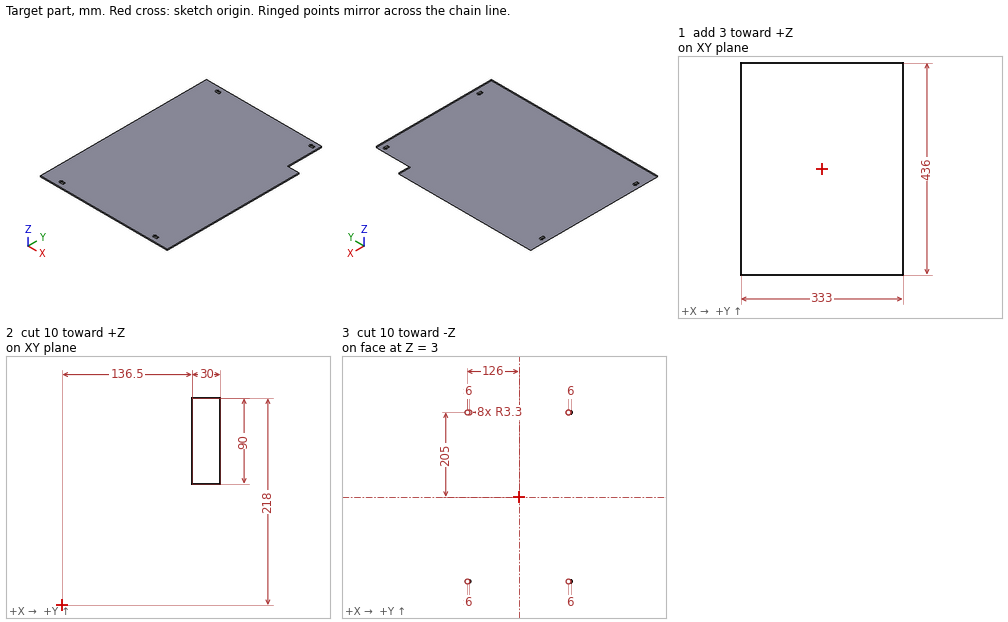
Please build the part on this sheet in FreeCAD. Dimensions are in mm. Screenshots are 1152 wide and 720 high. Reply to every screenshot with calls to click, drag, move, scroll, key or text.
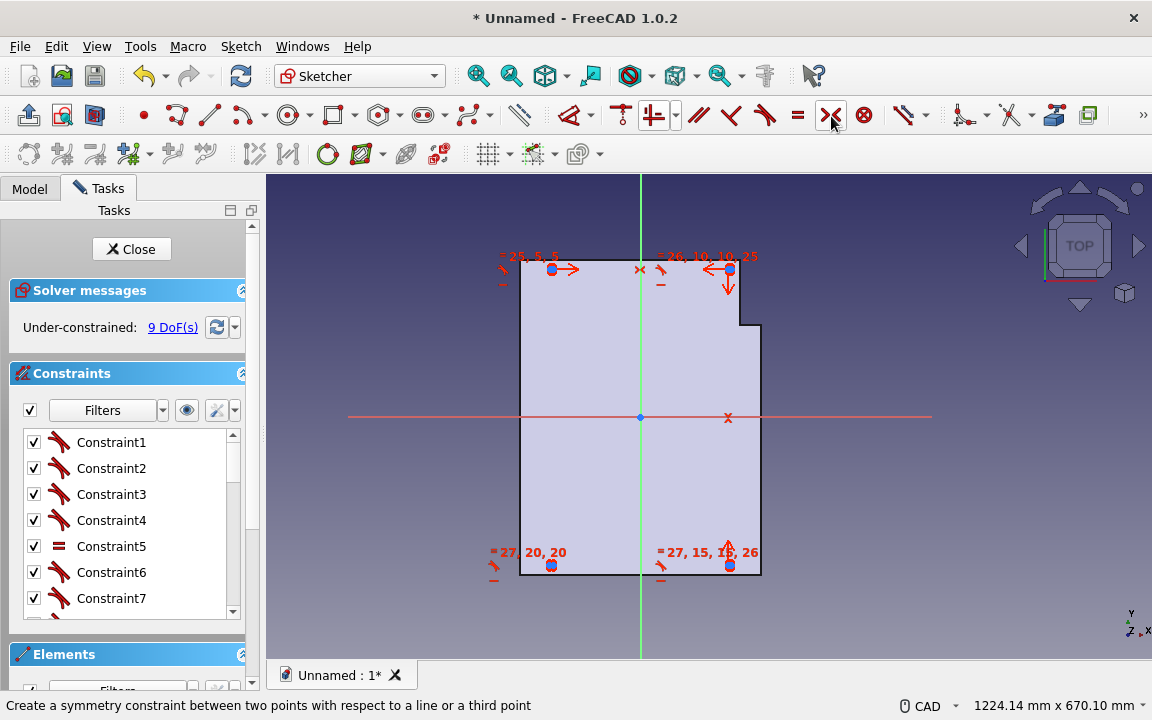
scroll(551, 269, up, 8)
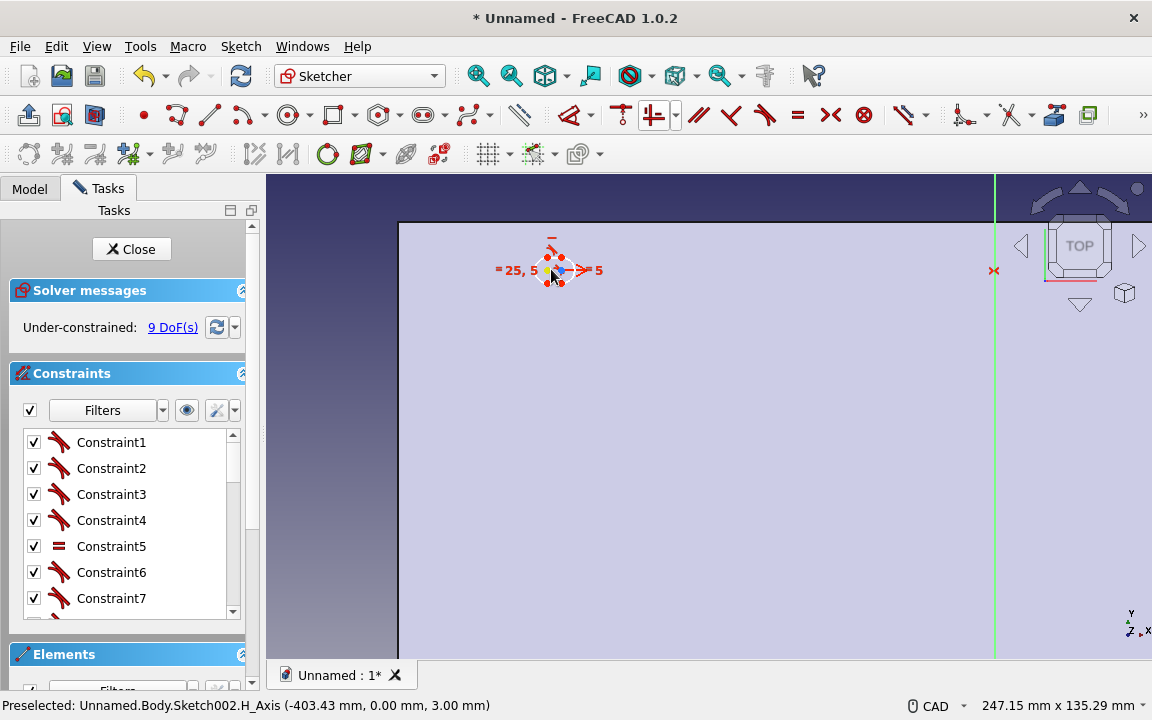
click(548, 270)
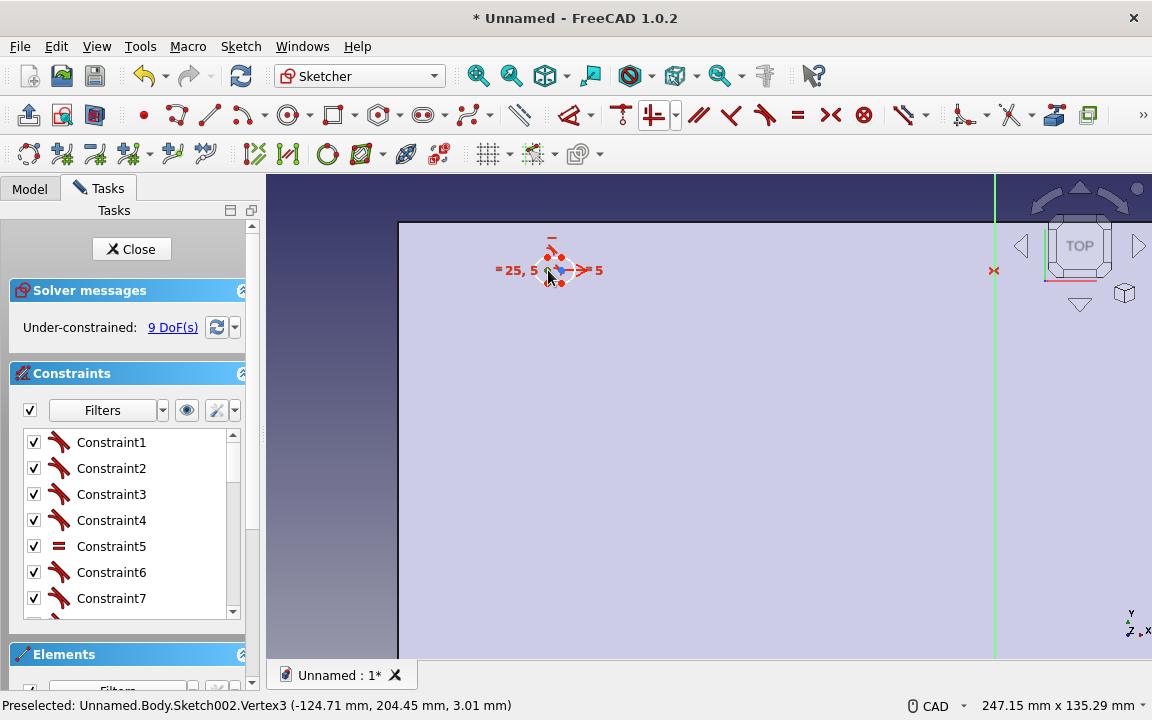
scroll(551, 268, down, 8)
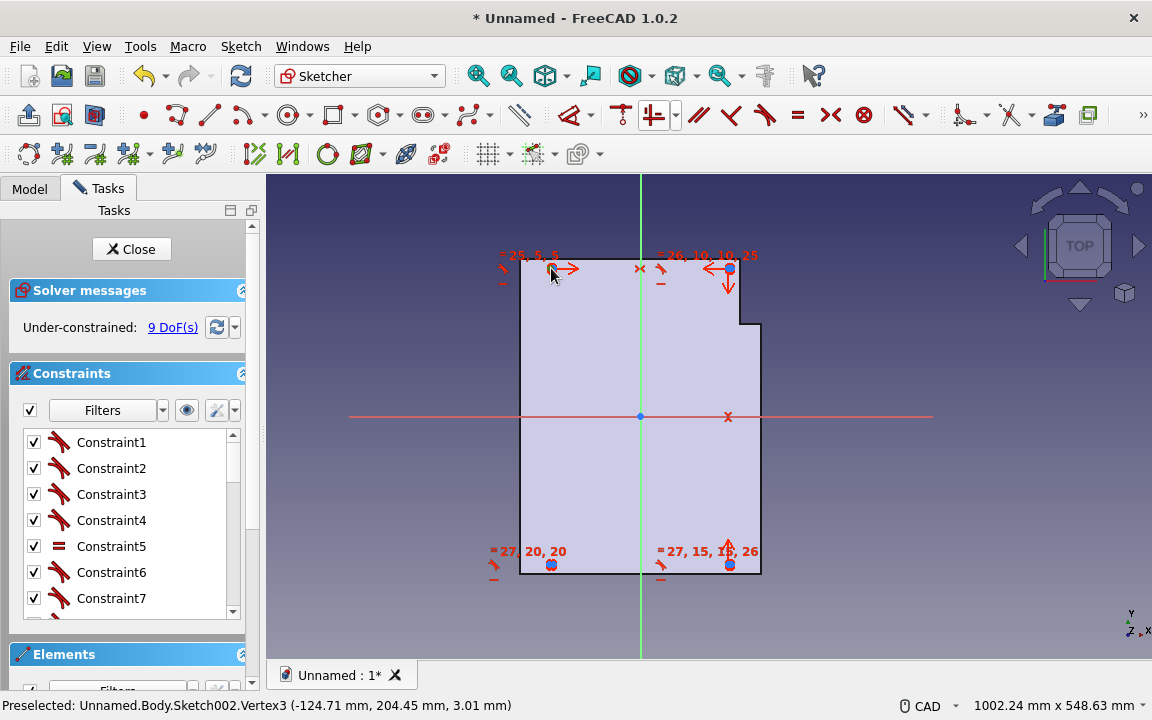
scroll(550, 565, up, 8)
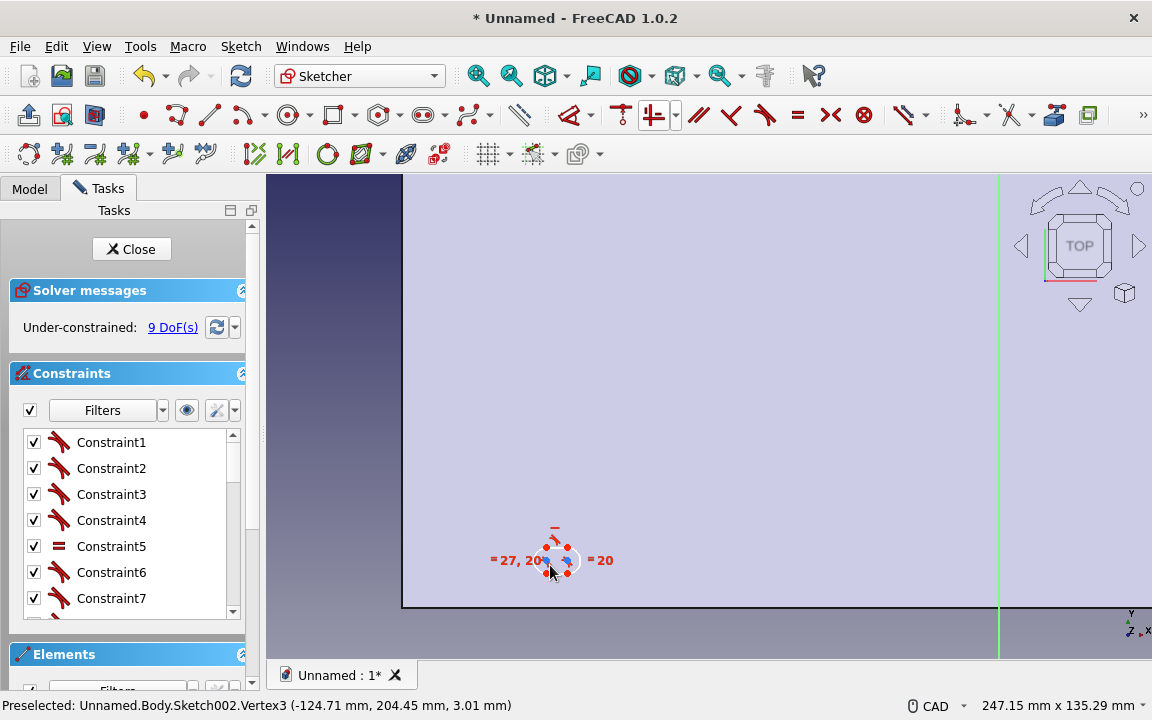
click(547, 561)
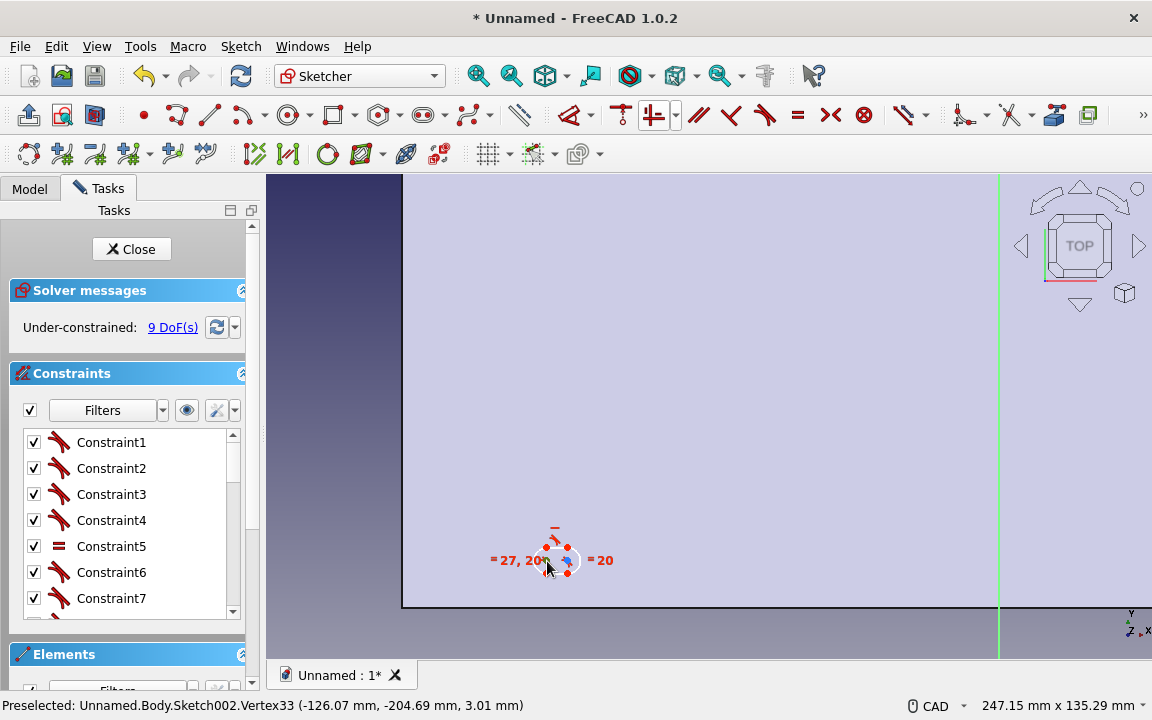
scroll(550, 566, down, 8)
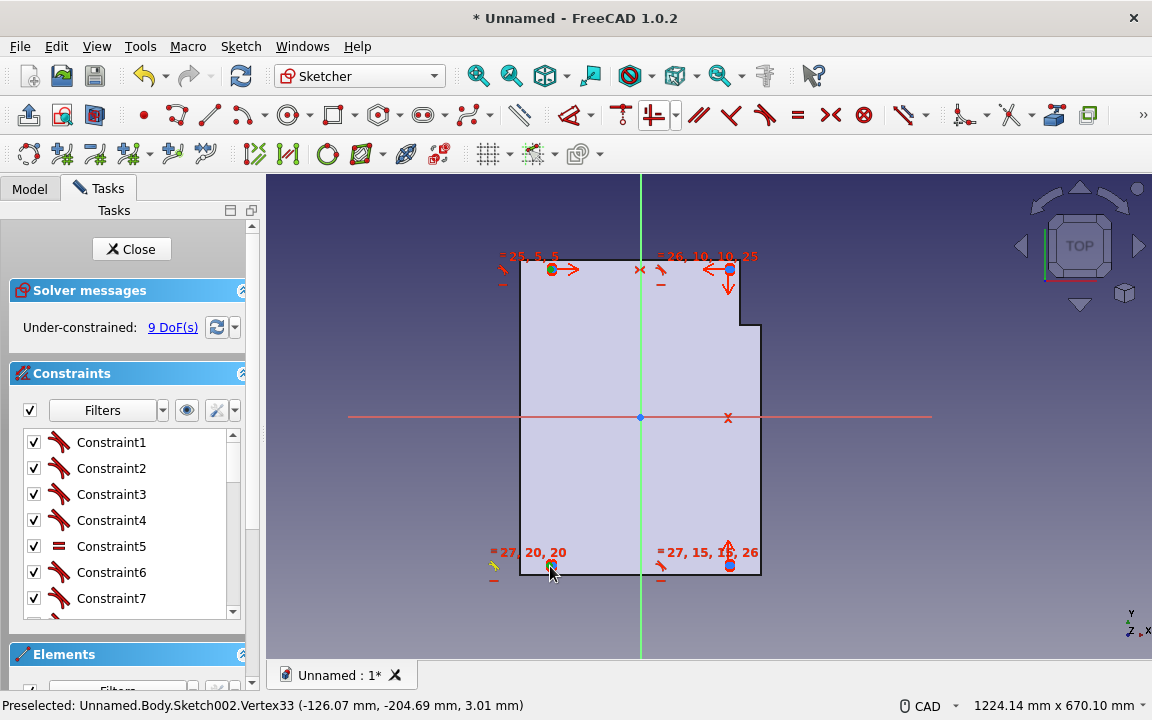
click(344, 417)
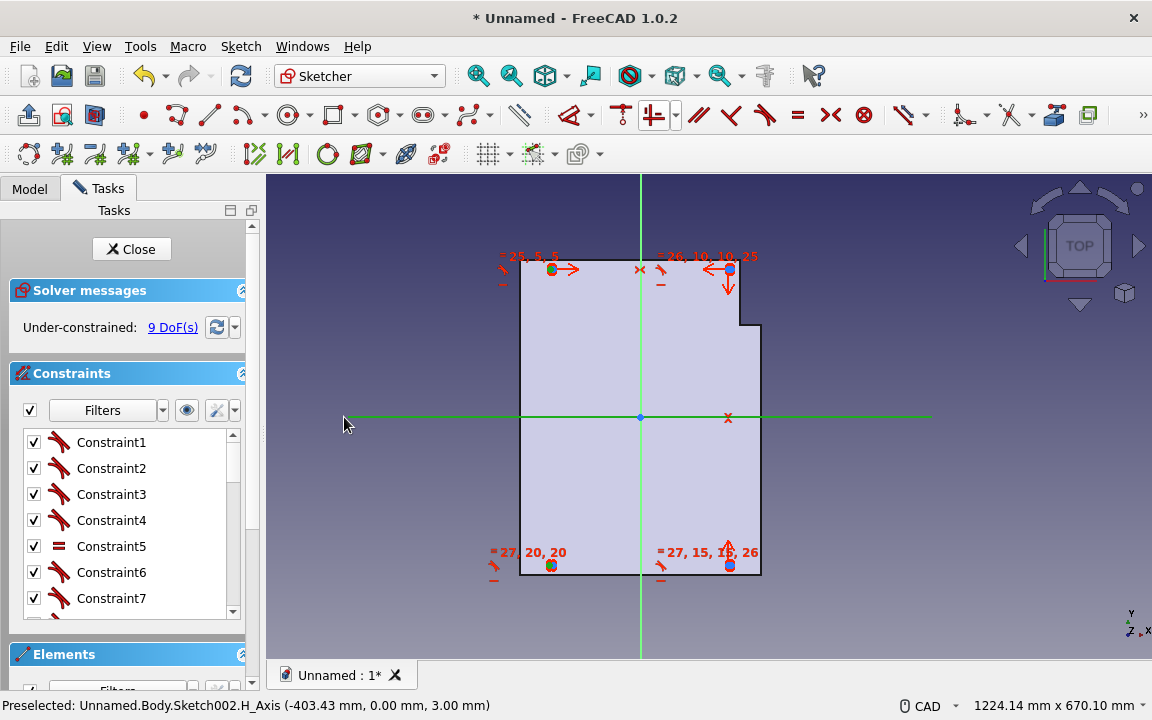
click(831, 116)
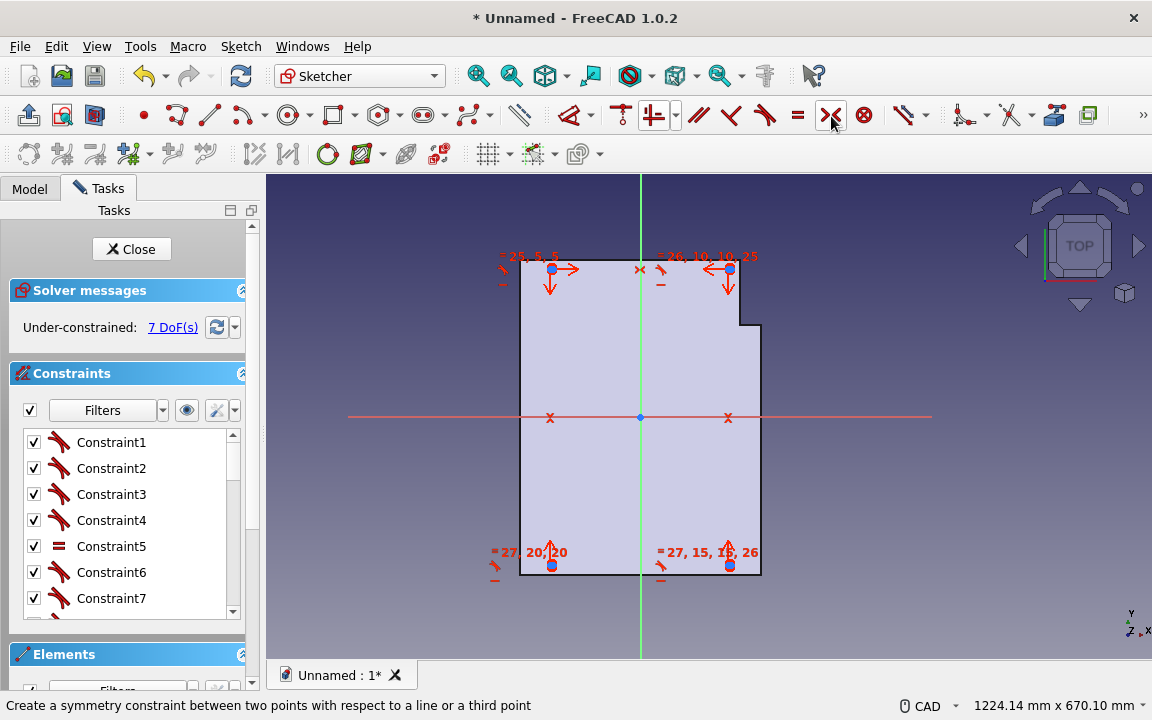
click(568, 116)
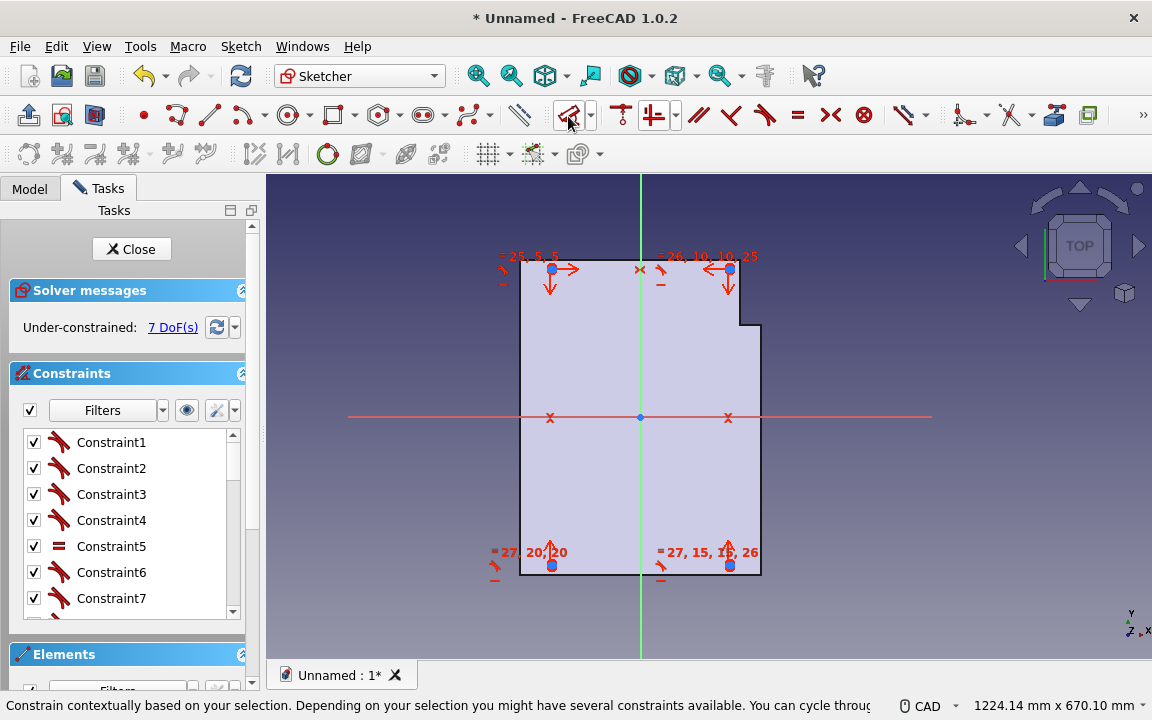
scroll(548, 269, up, 15)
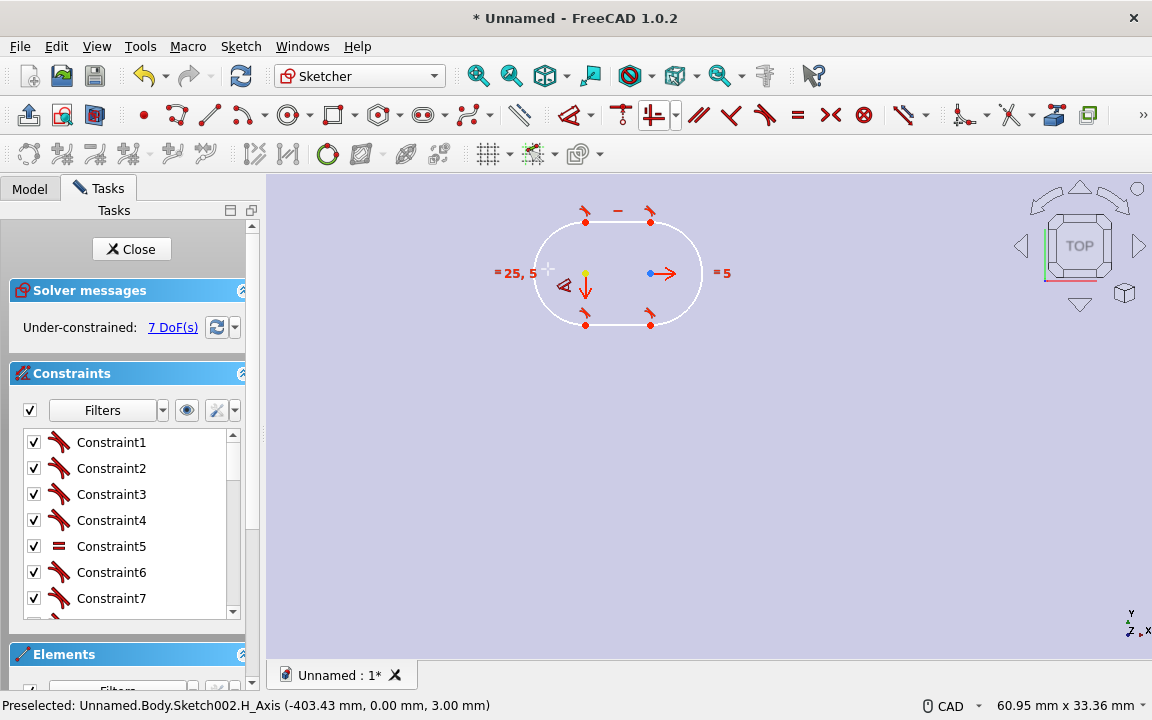
click(534, 274)
click(502, 274)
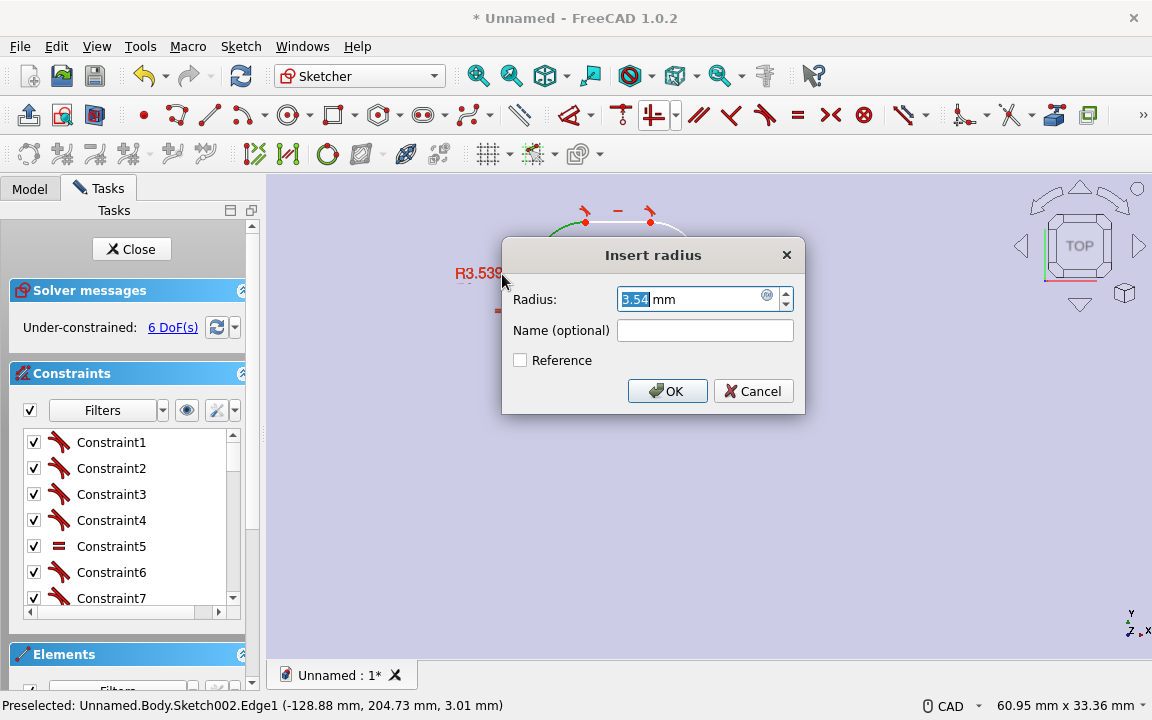
text(3.3)
key(Return)